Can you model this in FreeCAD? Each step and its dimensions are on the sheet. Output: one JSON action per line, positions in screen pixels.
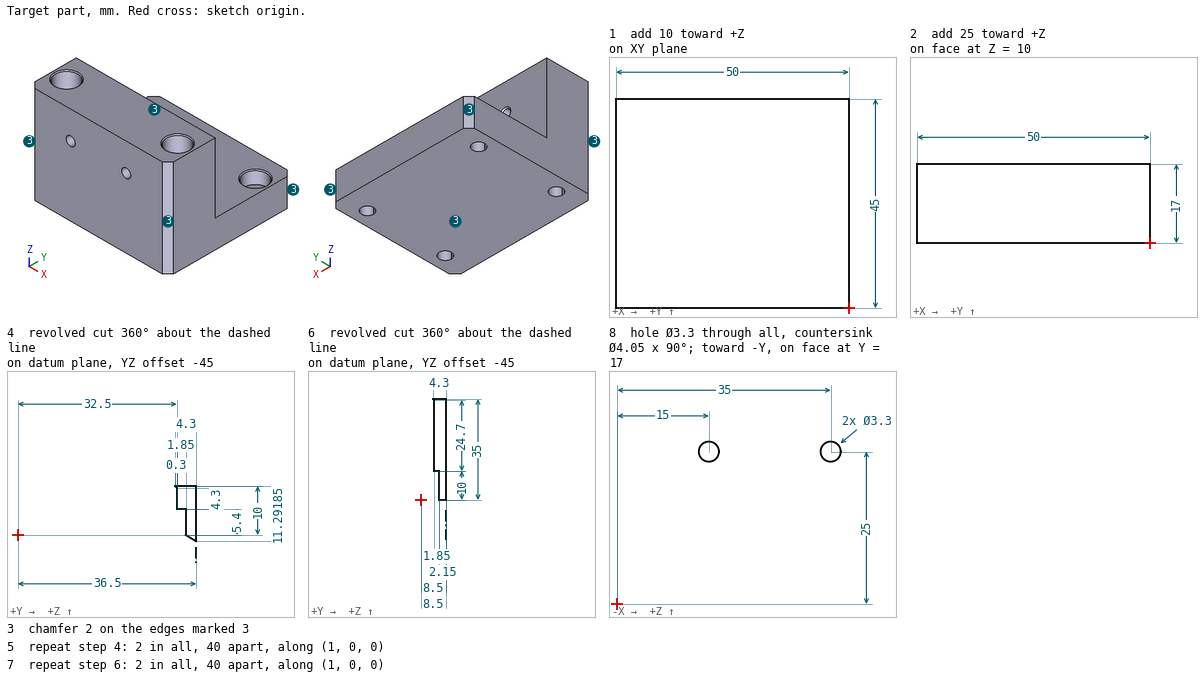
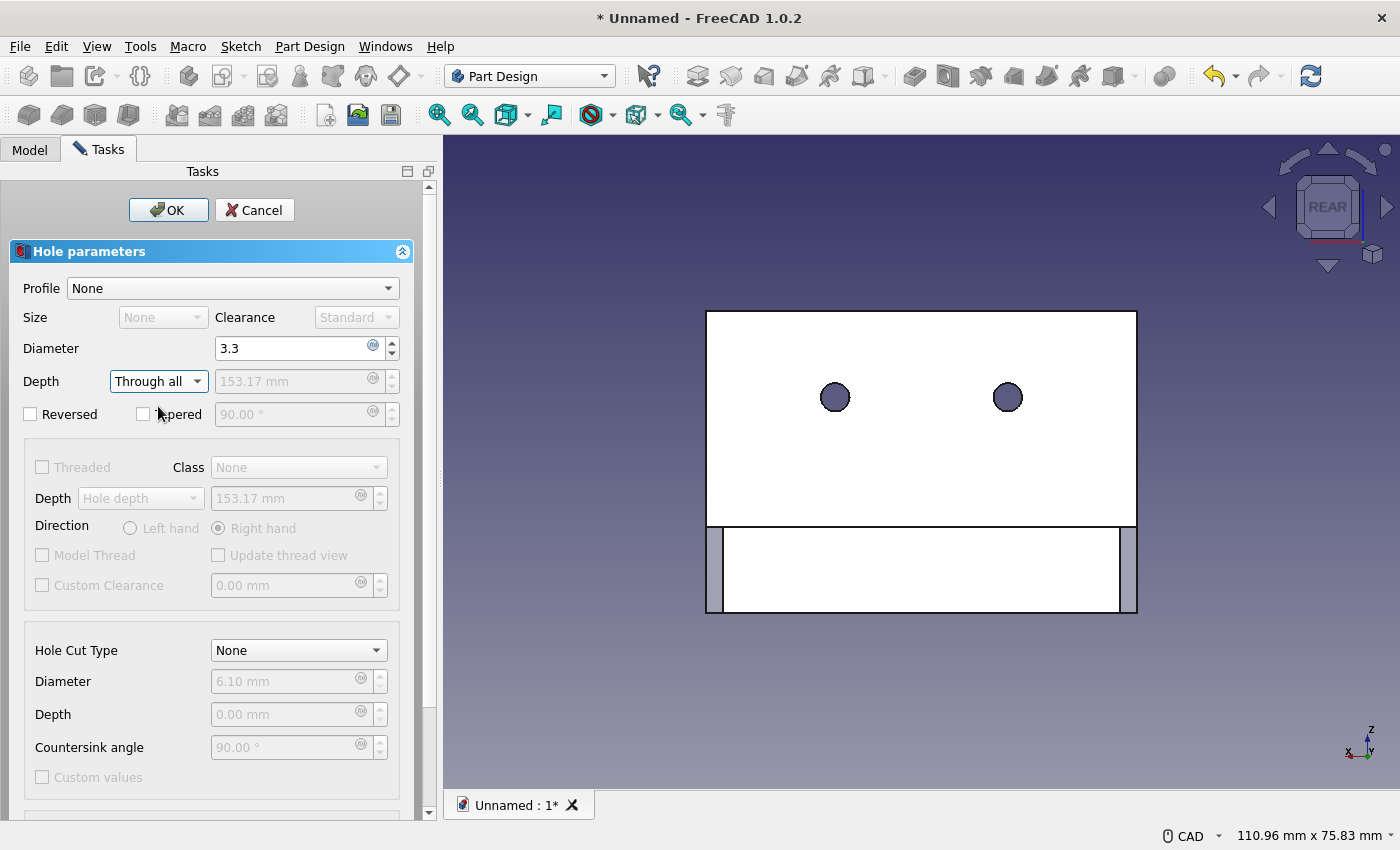
{"action": "left_click", "coordinate": [300, 650]}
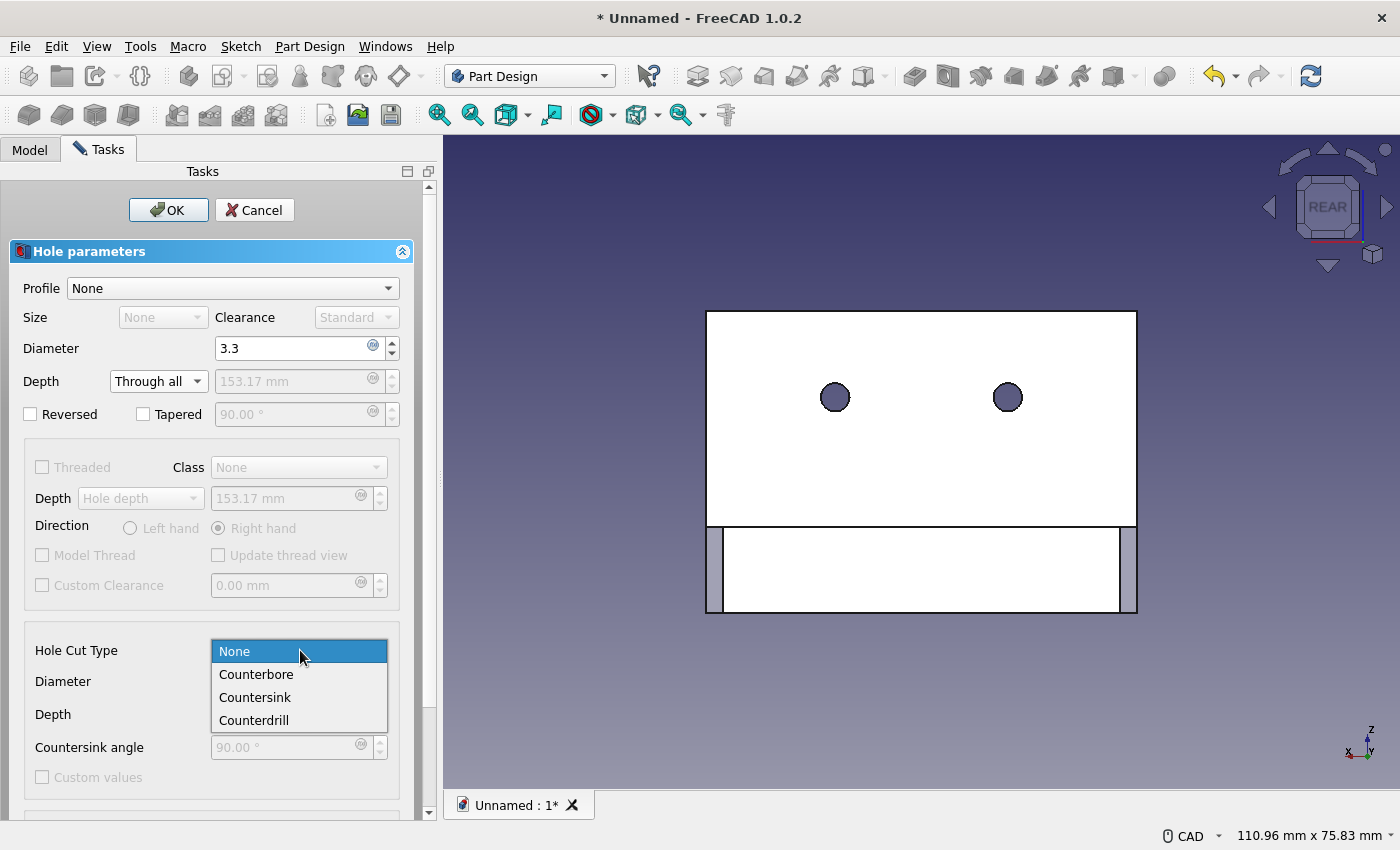
{"action": "left_click", "coordinate": [298, 698]}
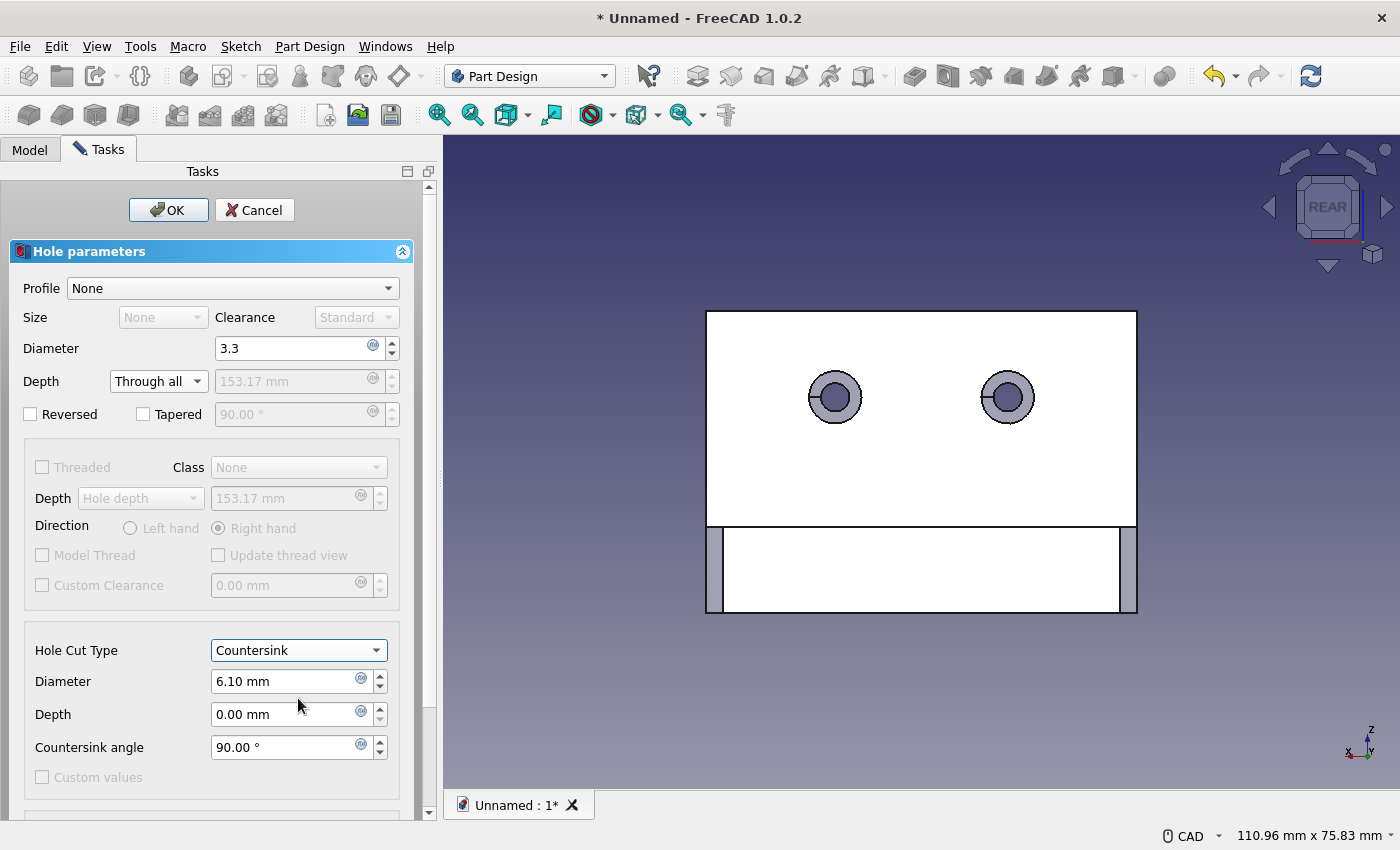
{"action": "triple_click", "coordinate": [292, 682]}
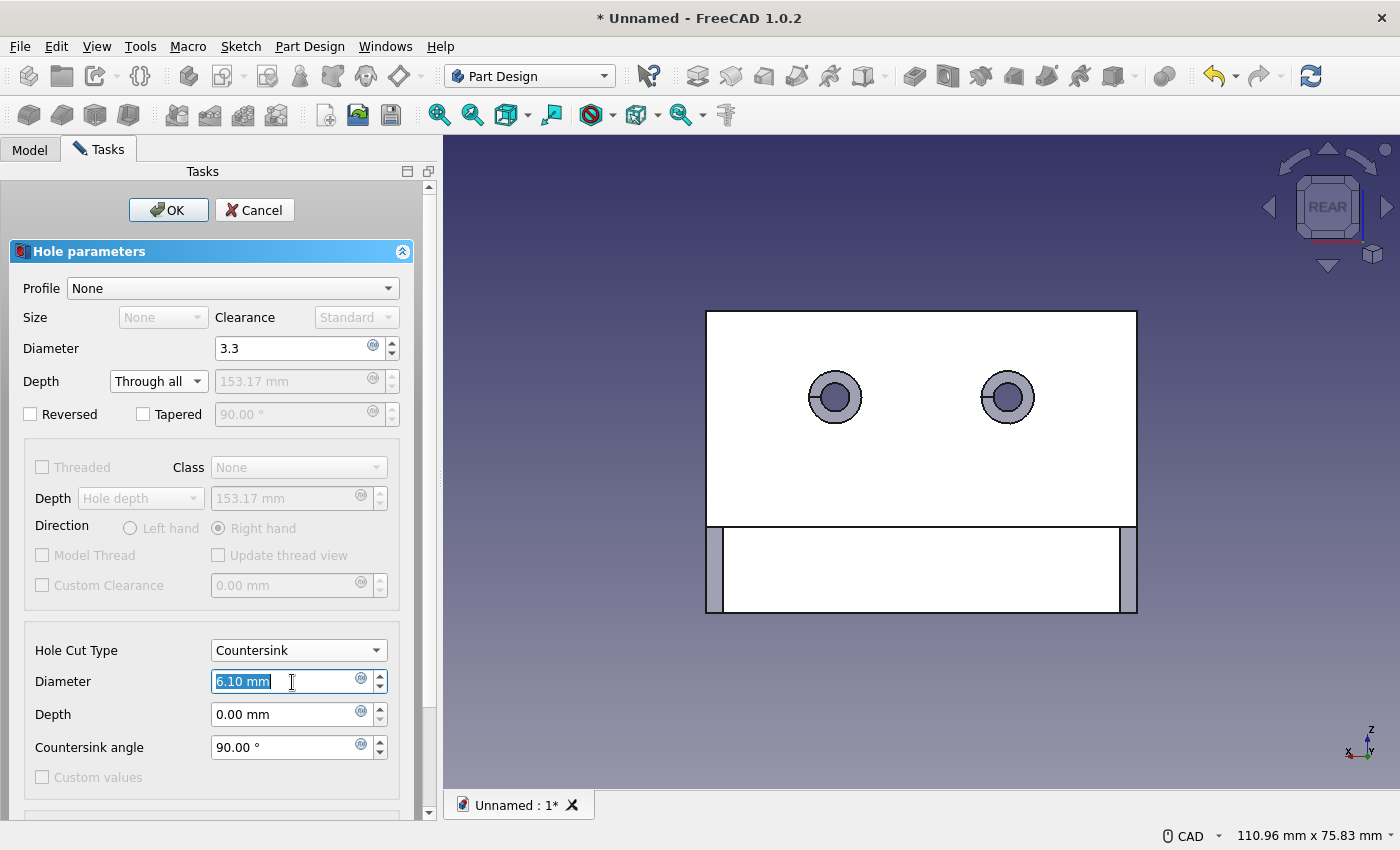
{"action": "type", "text": "4.05"}
{"action": "key", "text": "Tab"}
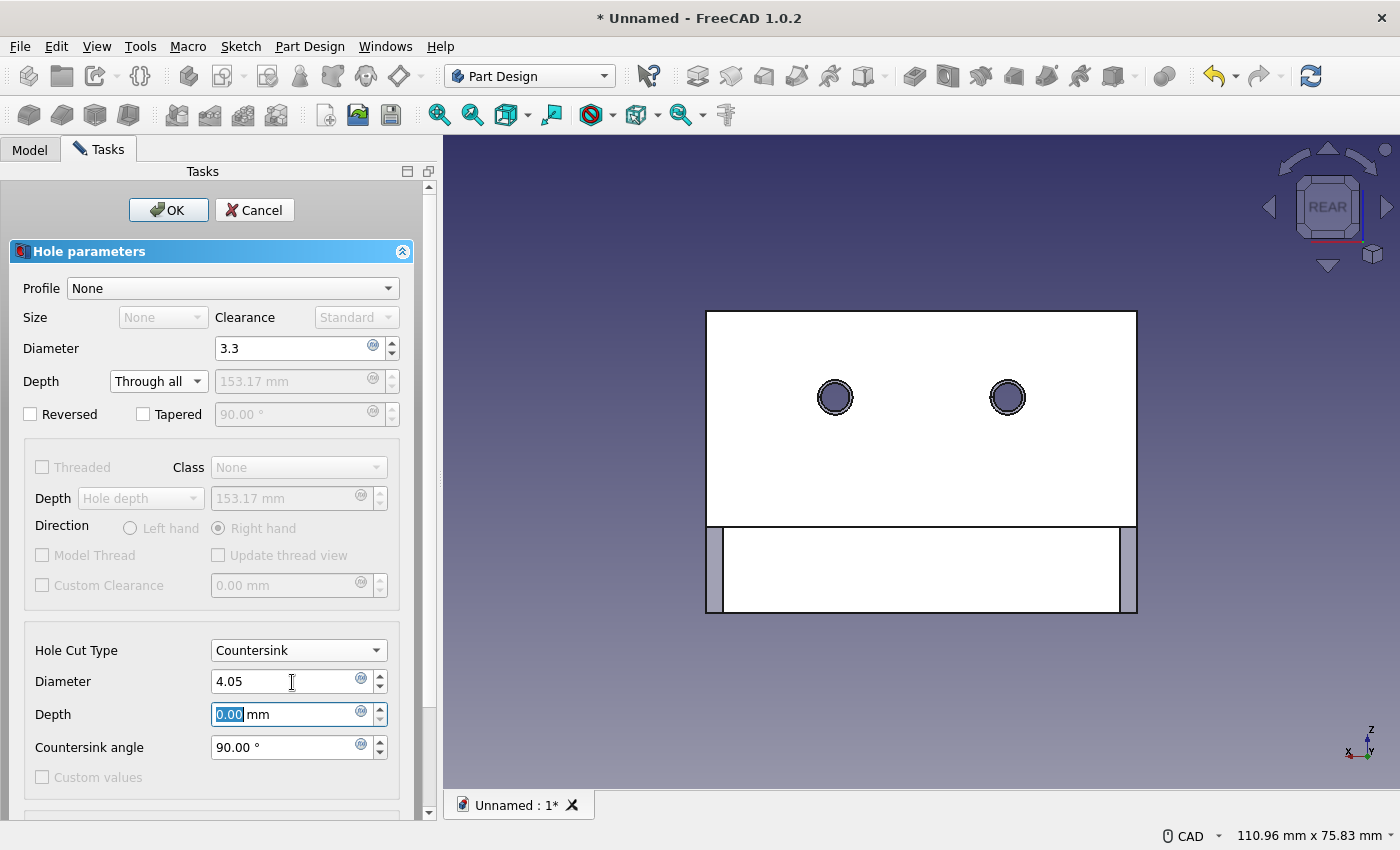
{"action": "left_click", "coordinate": [169, 210]}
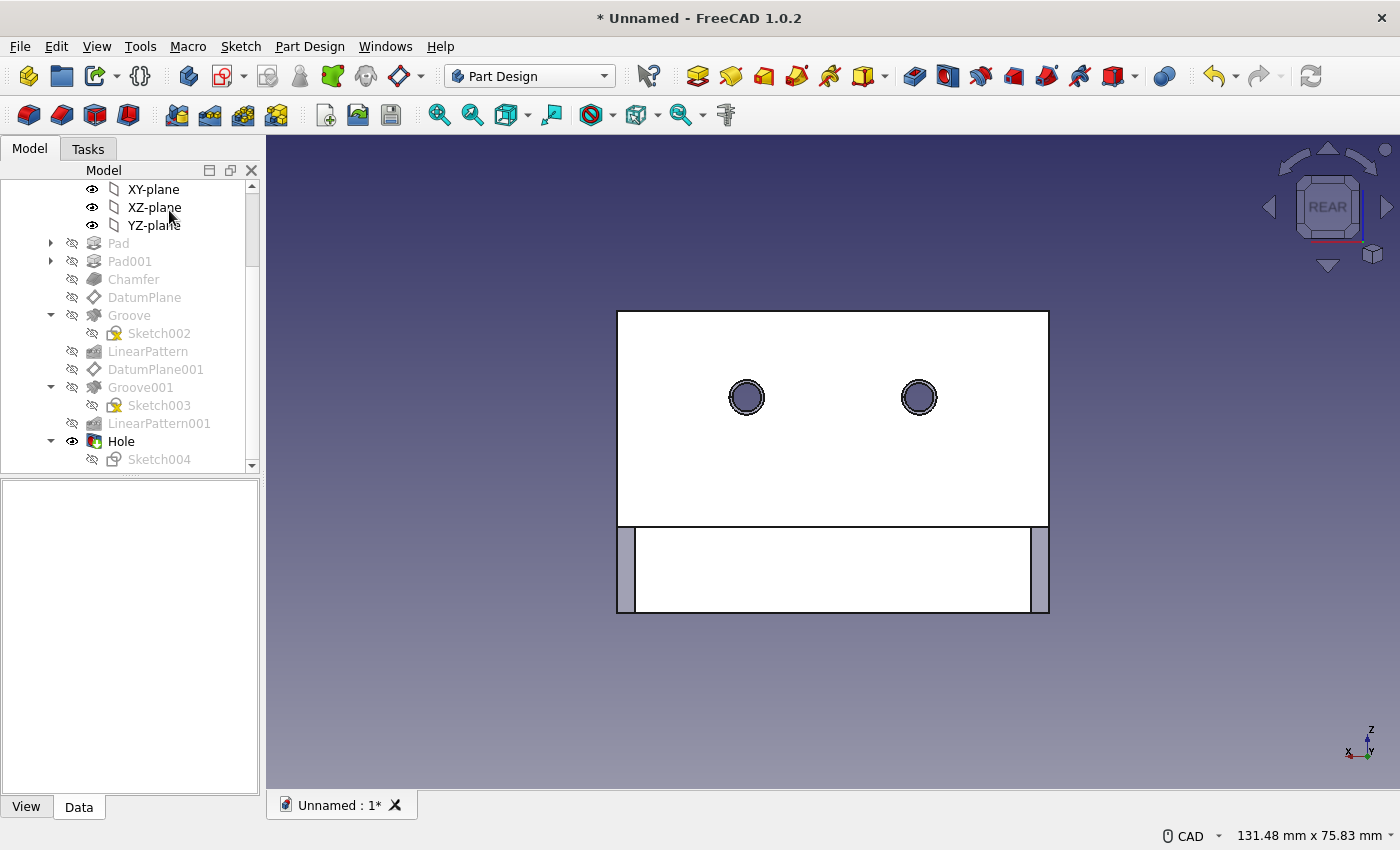
{"action": "key", "text": "0"}